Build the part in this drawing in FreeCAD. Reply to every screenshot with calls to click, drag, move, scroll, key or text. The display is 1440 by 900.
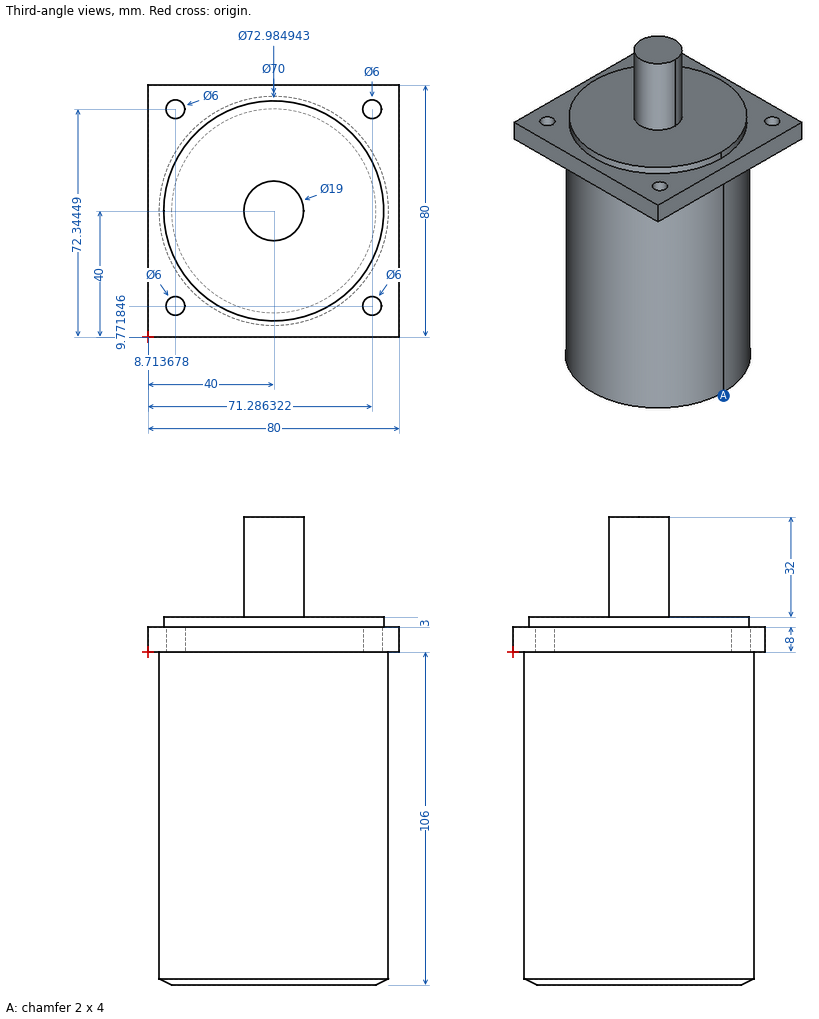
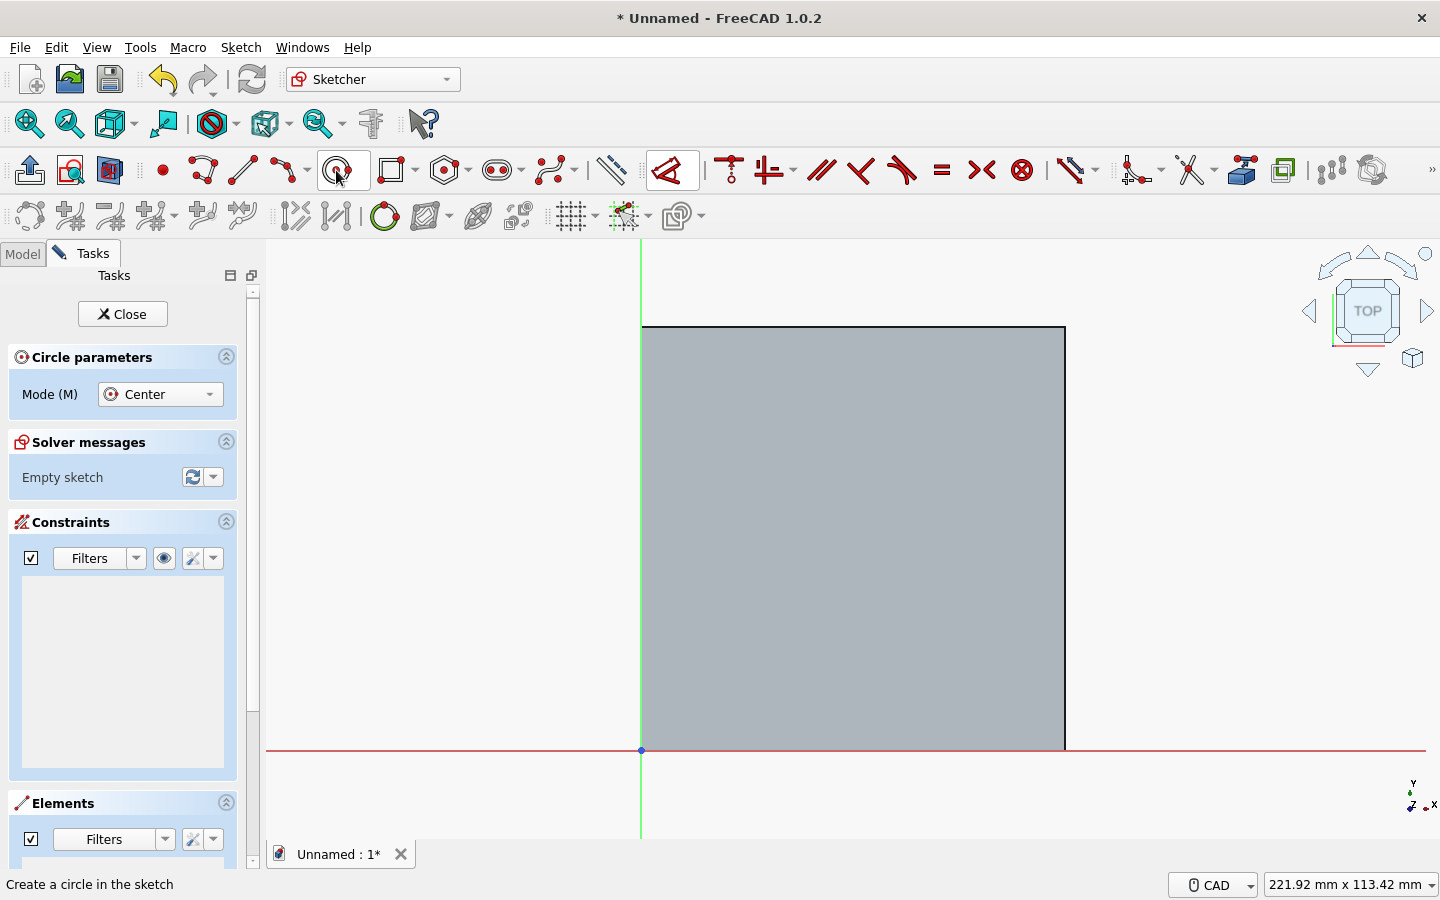
click(853, 539)
move(984, 408)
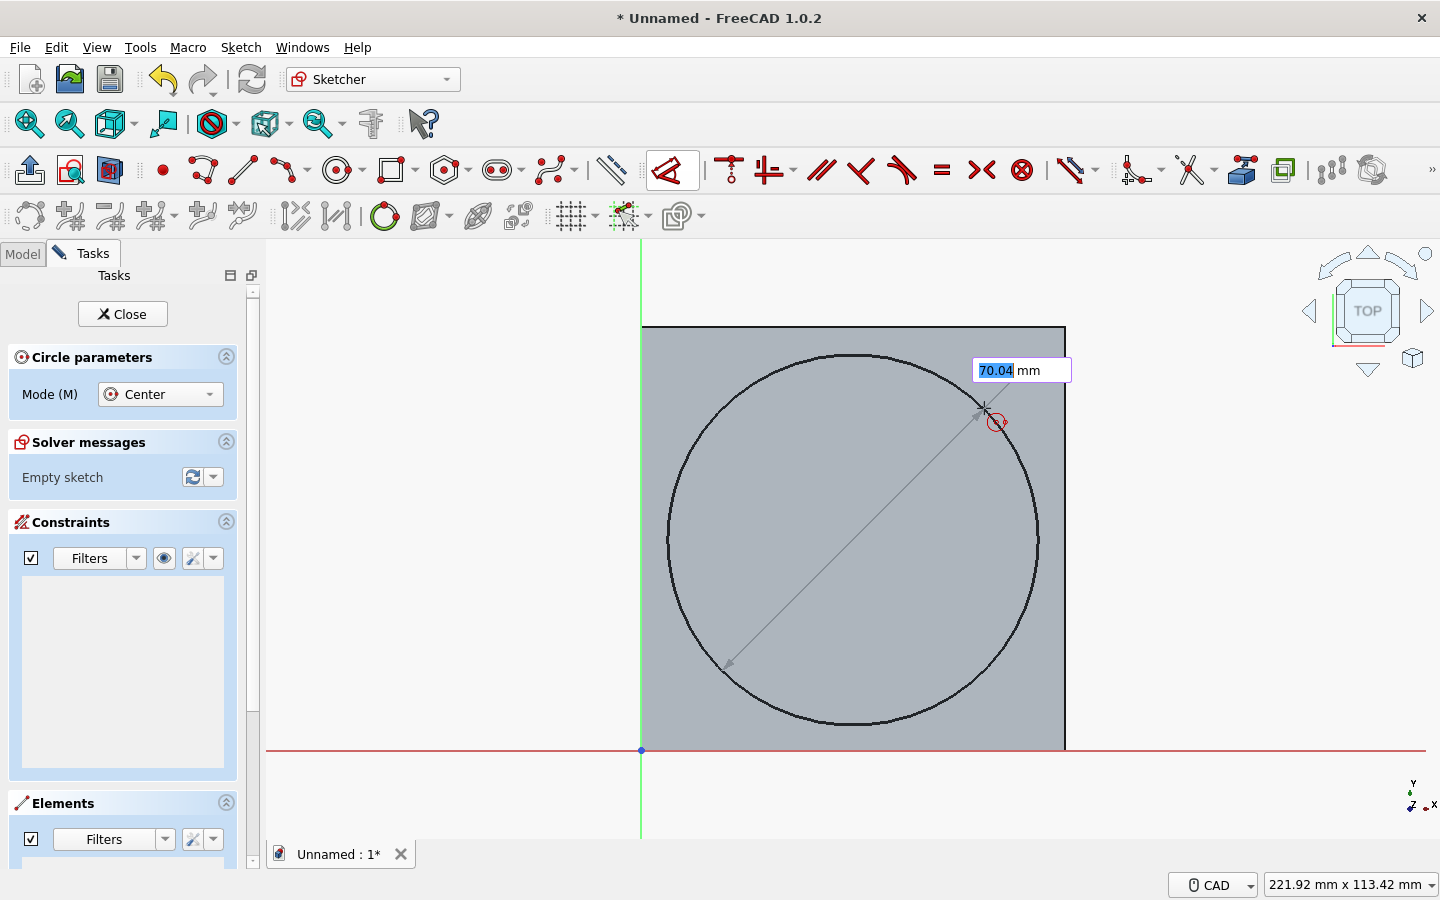
text(70)
key(Return)
key(Escape)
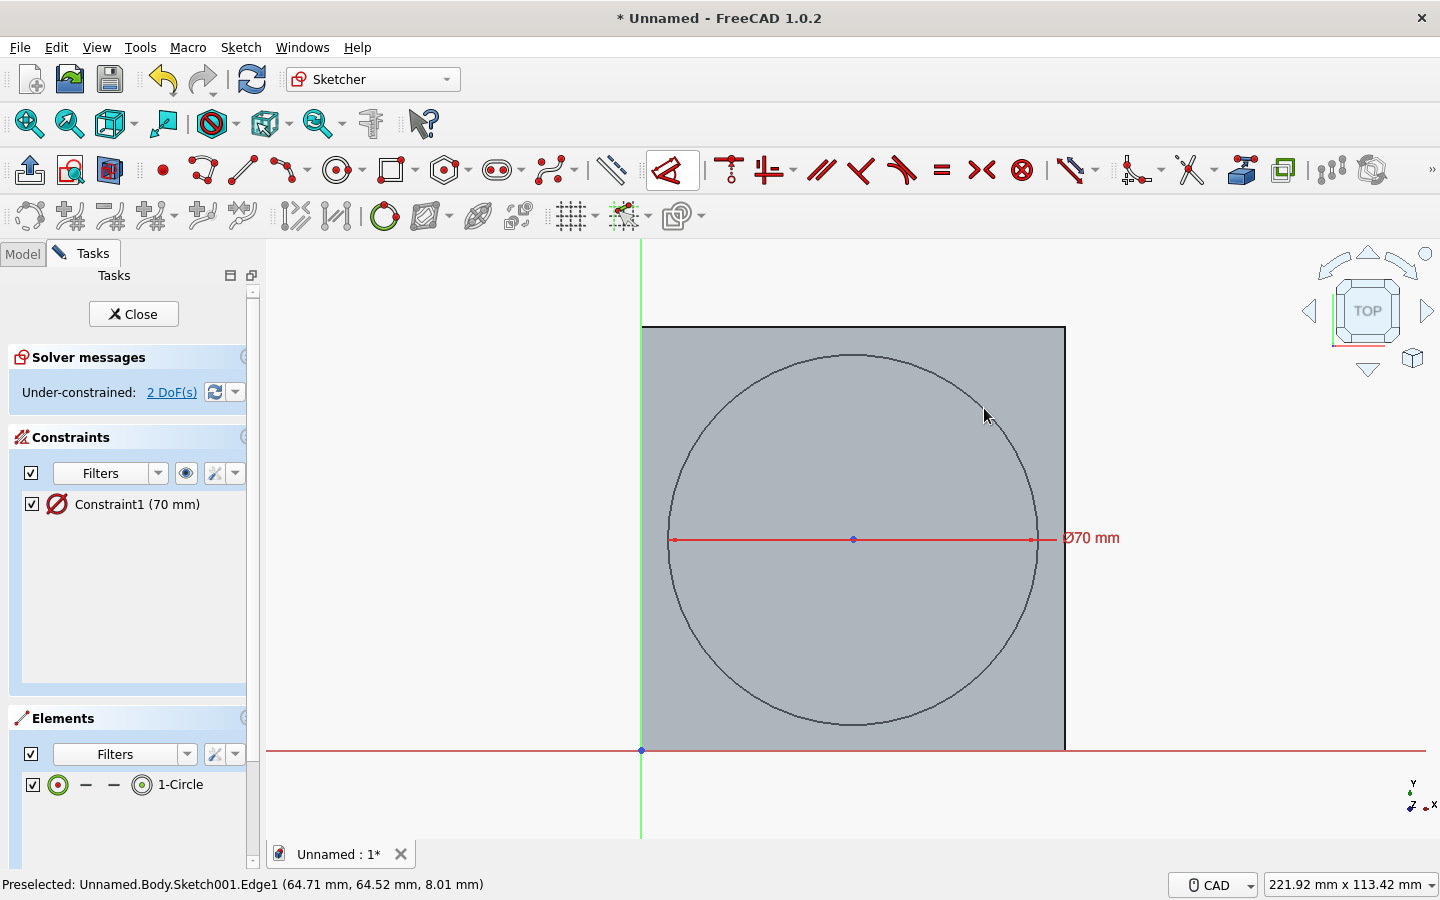
click(666, 170)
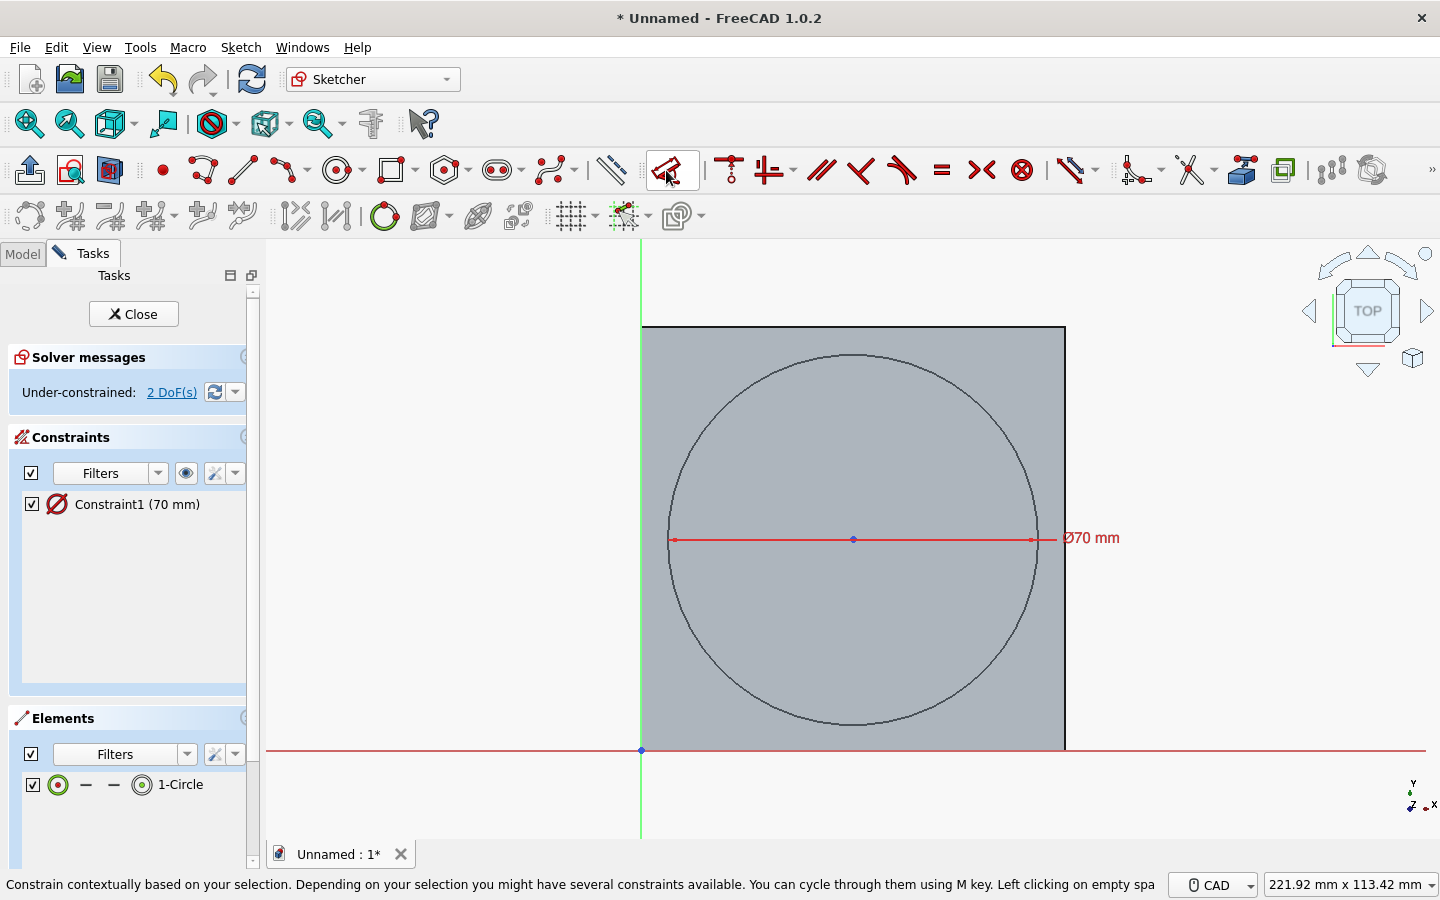
click(853, 540)
click(747, 785)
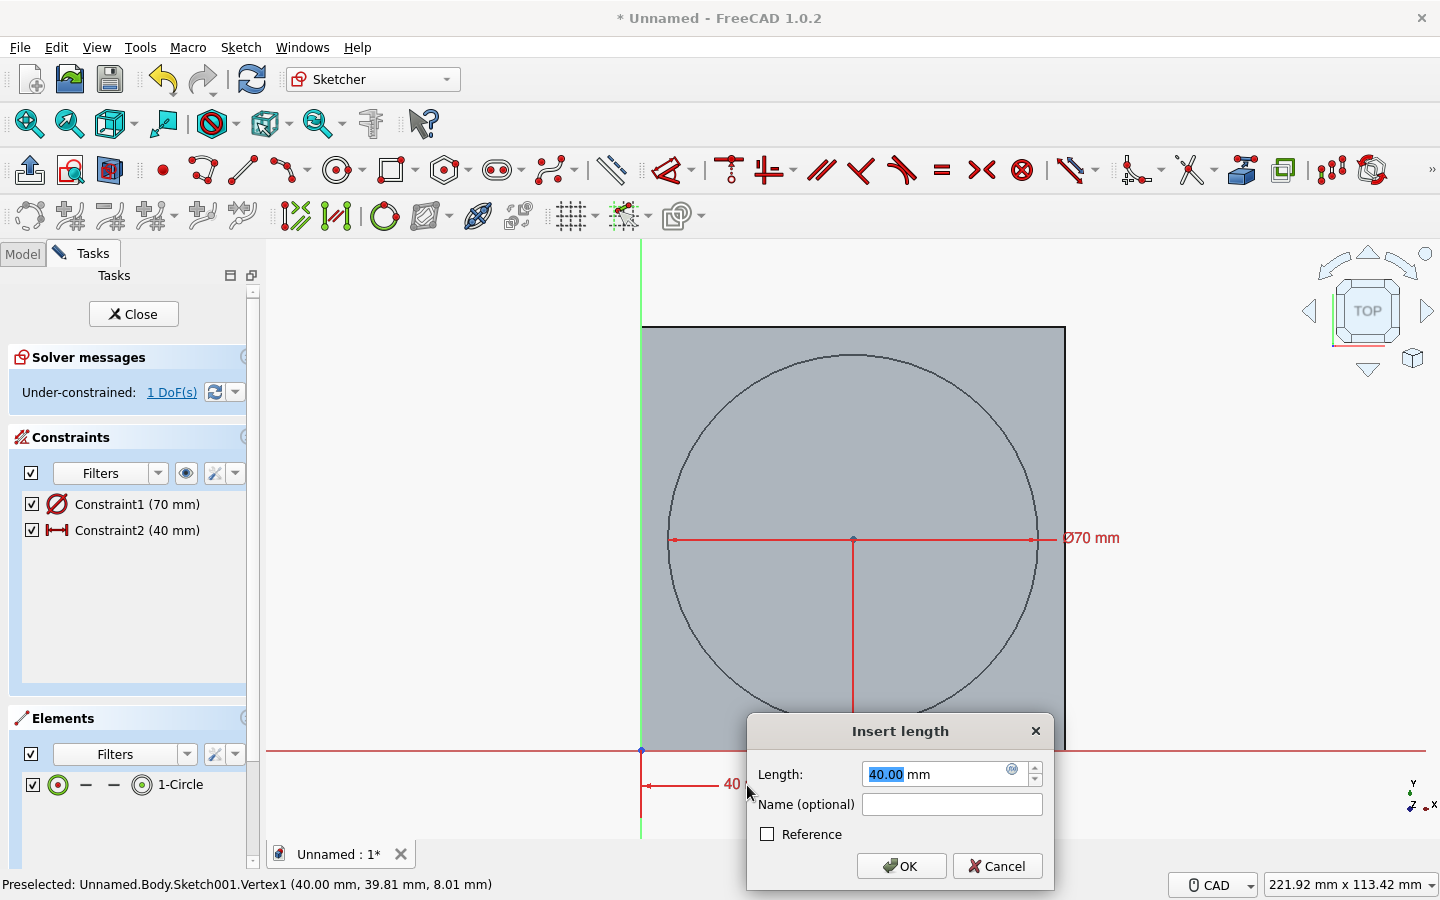
text(40)
key(Return)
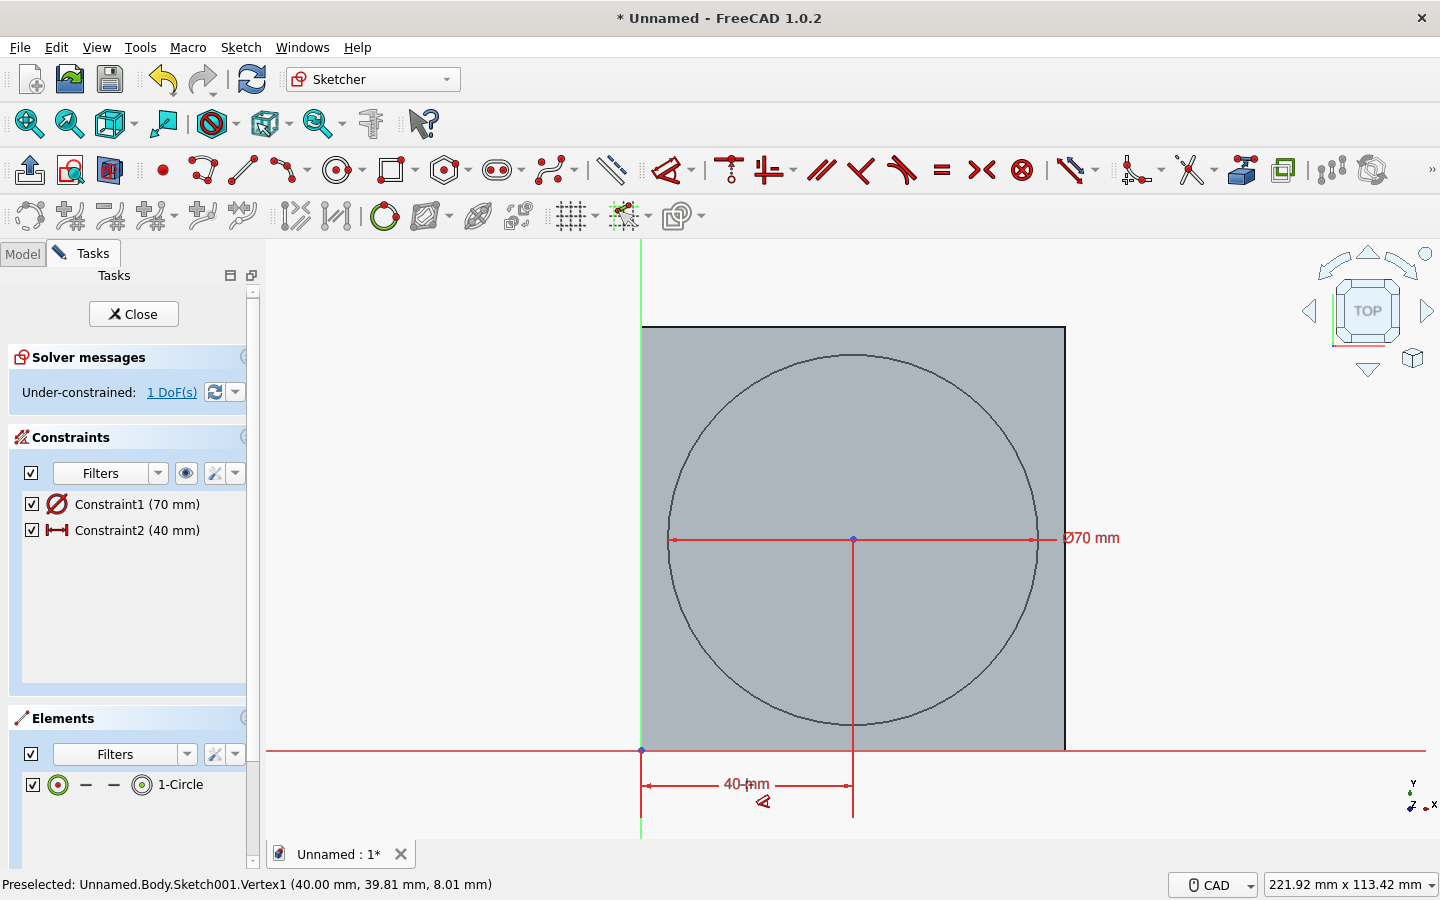
click(853, 540)
click(607, 645)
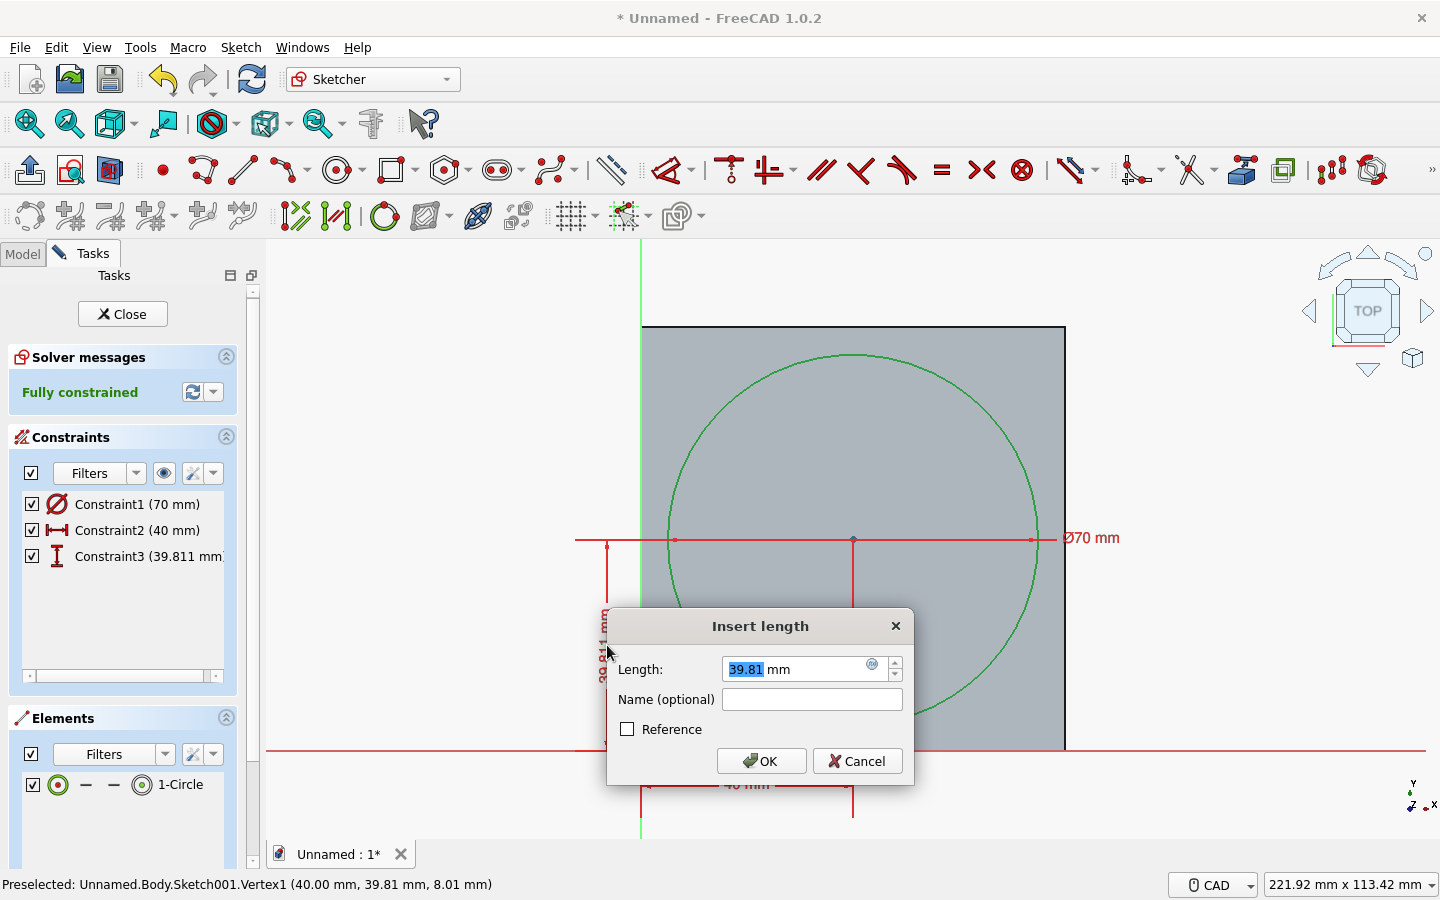
text(40)
key(Return)
key(Escape)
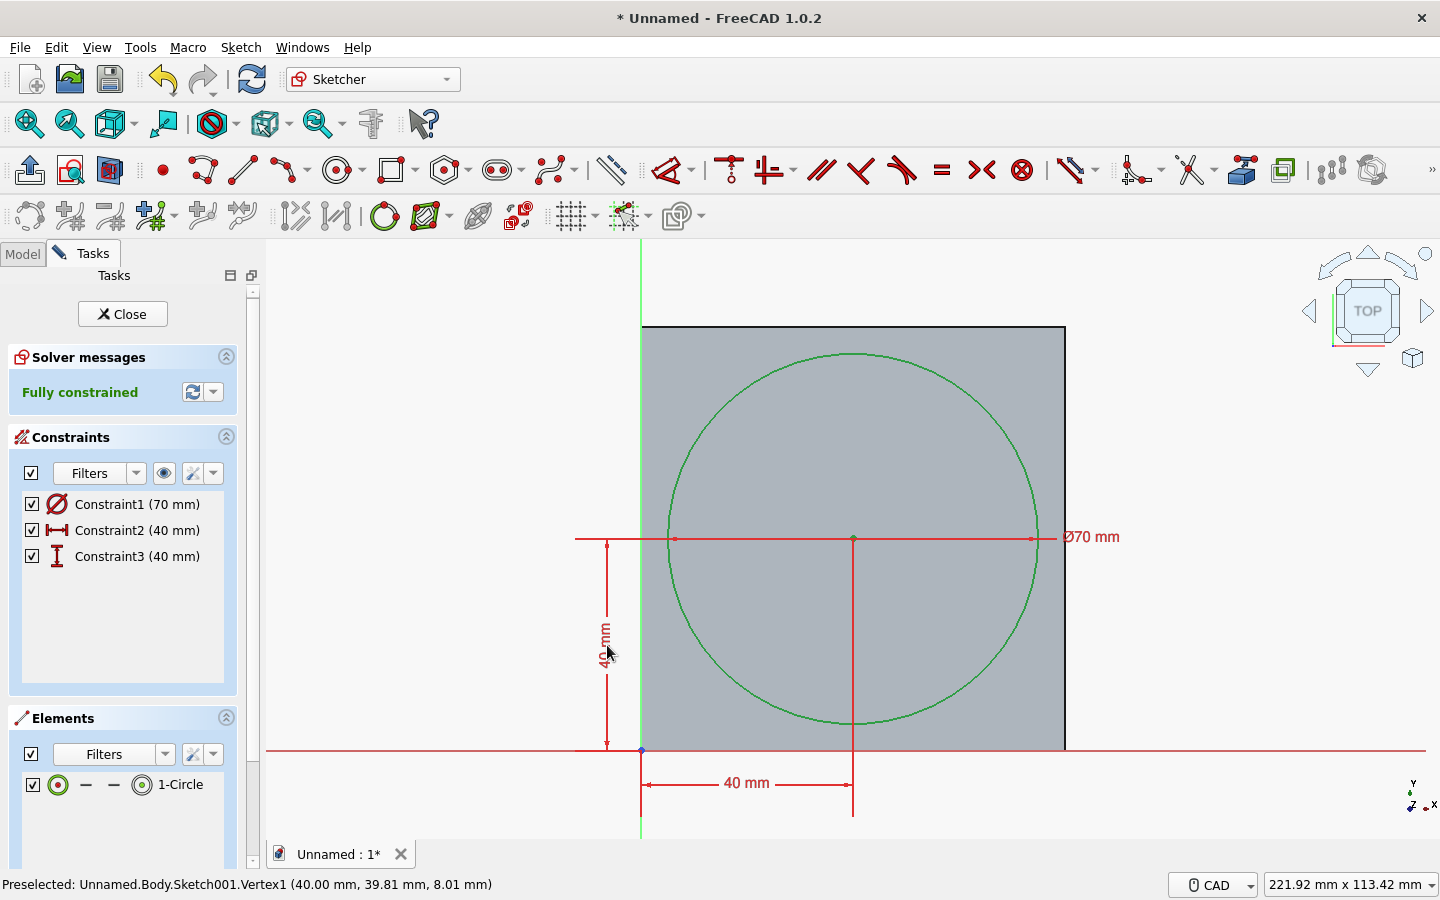
click(123, 314)